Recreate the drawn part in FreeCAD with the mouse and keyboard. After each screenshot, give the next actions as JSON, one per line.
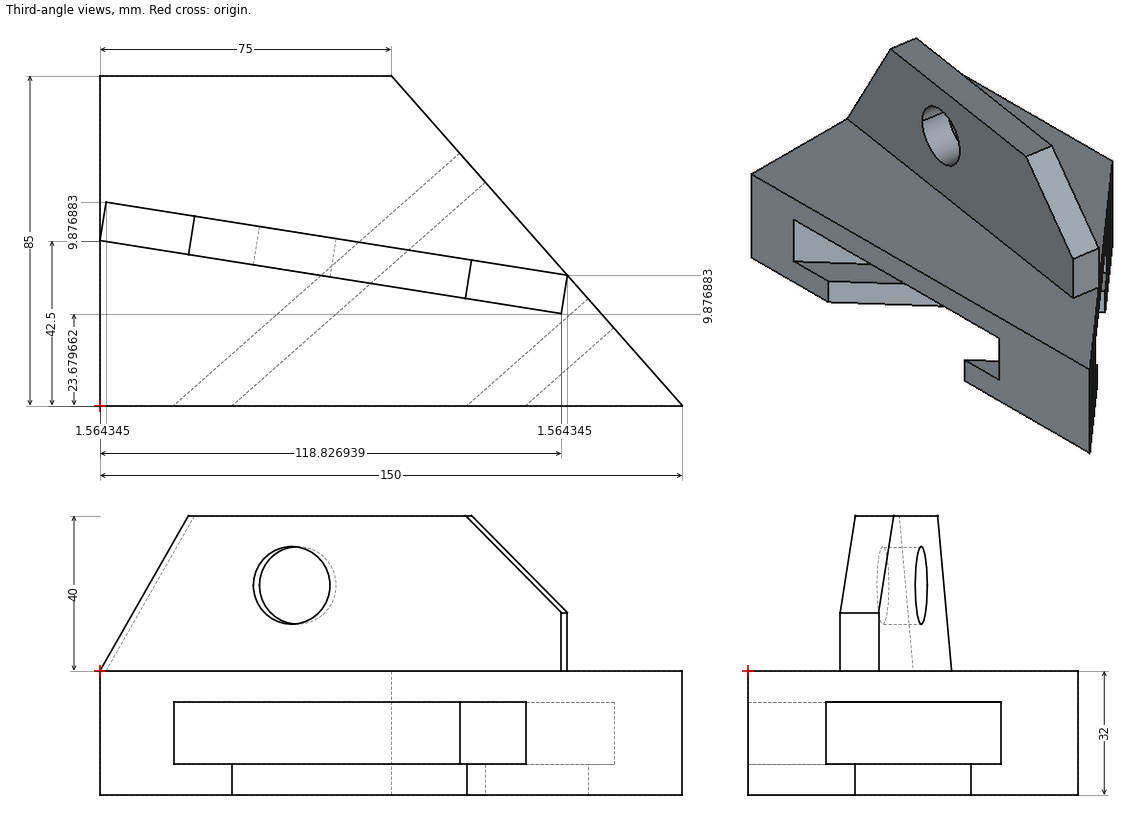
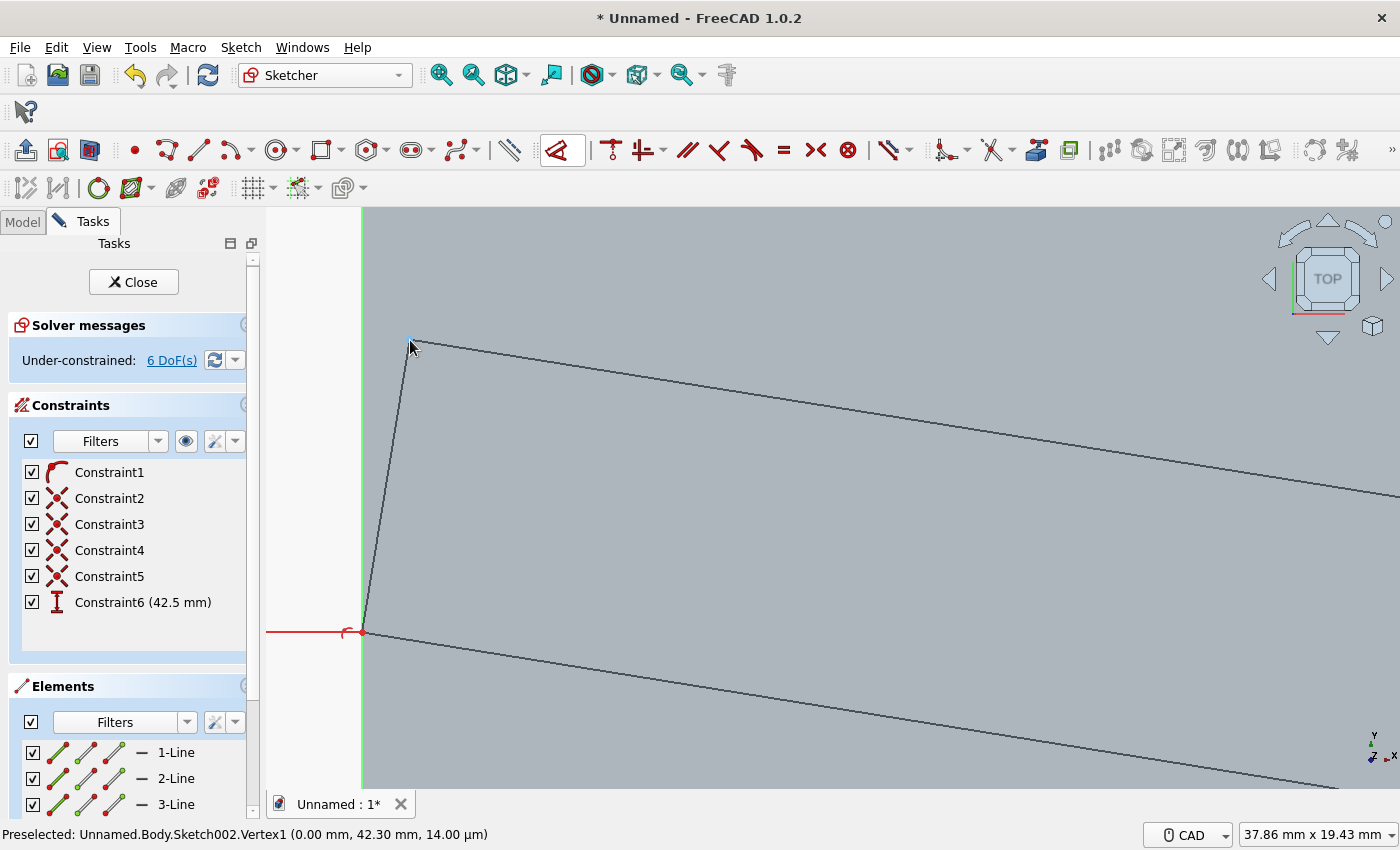
{"action": "left_click", "coordinate": [410, 340]}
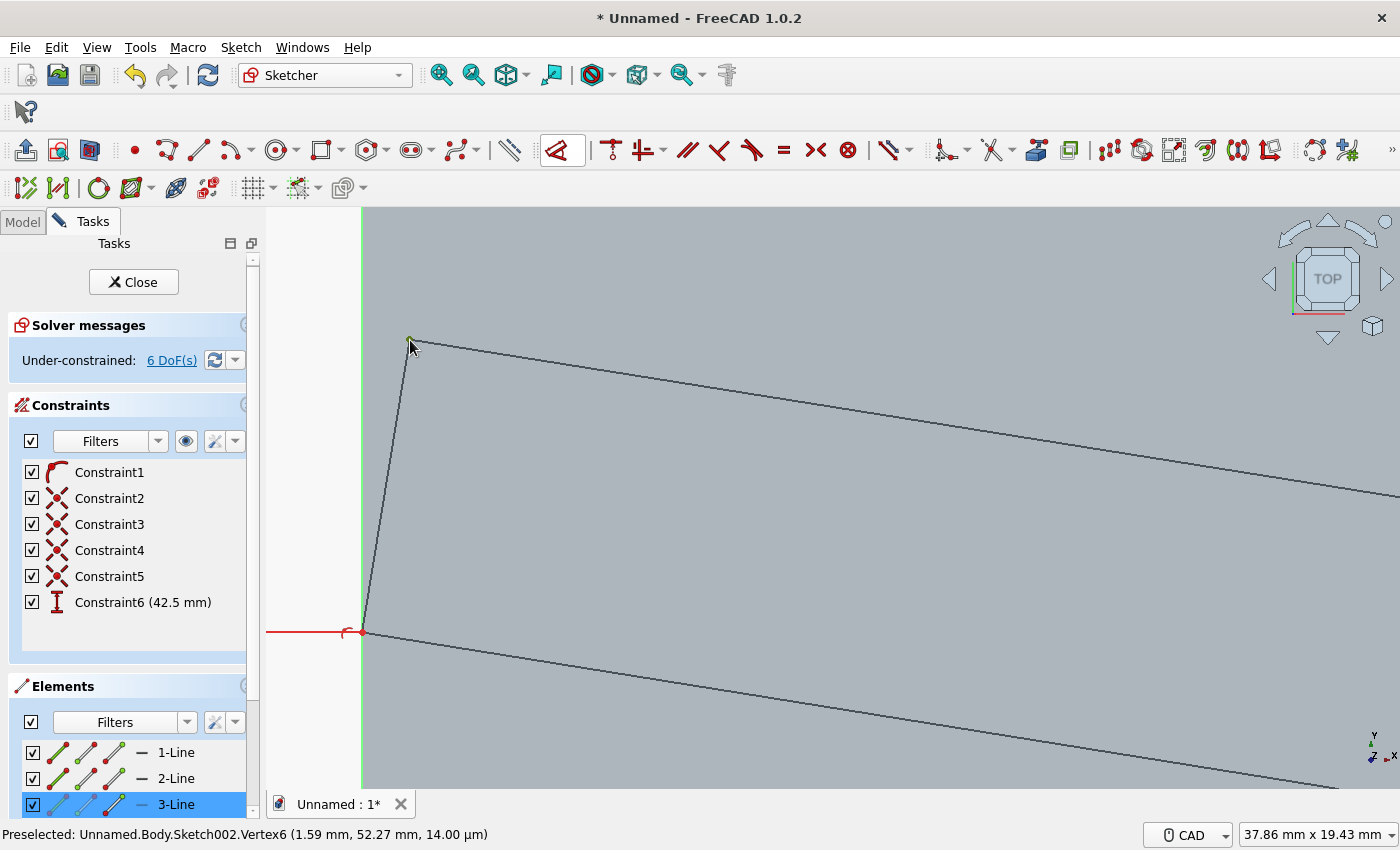
{"action": "key", "text": "l"}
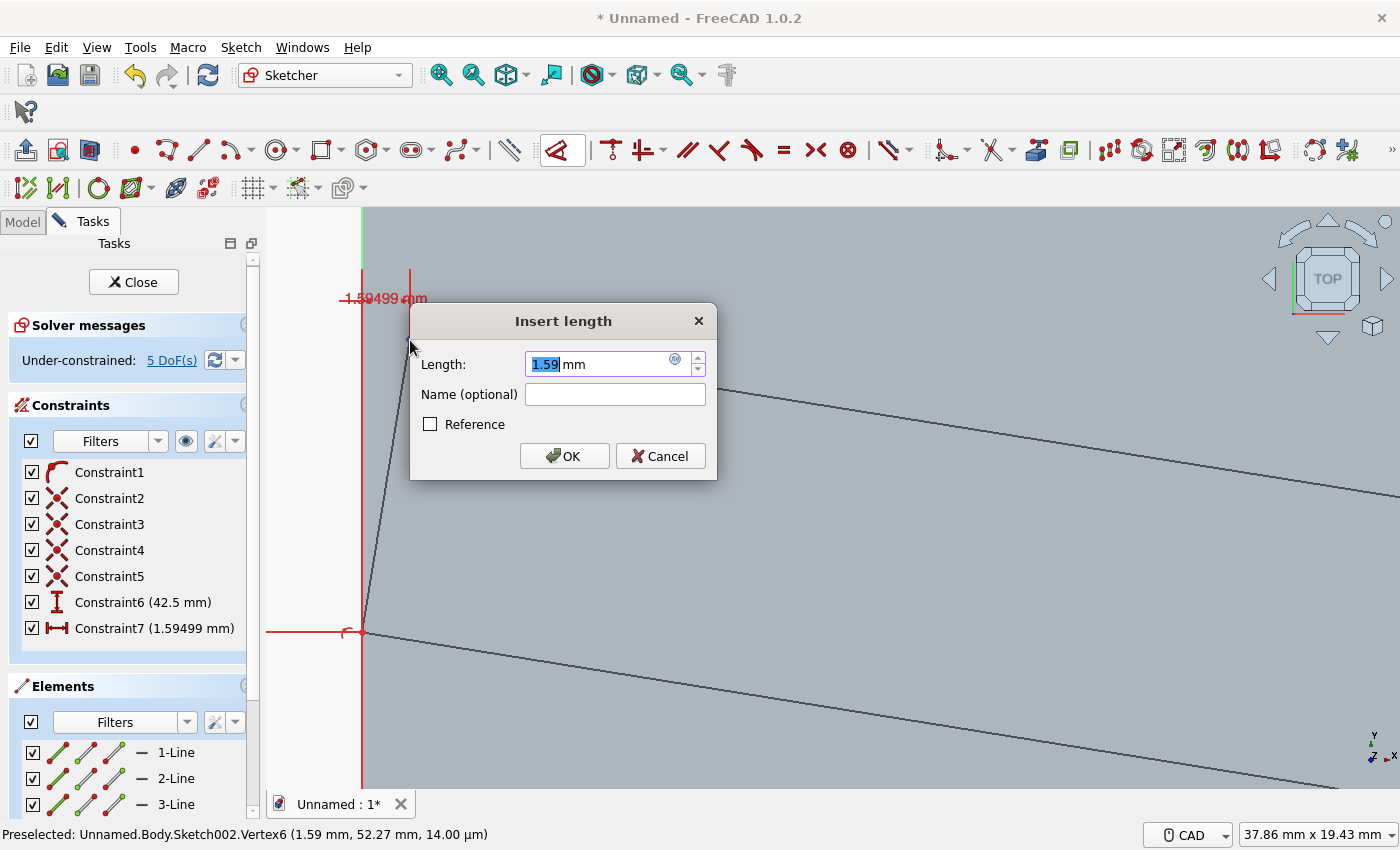
{"action": "type", "text": "1.564345"}
{"action": "key", "text": "Return"}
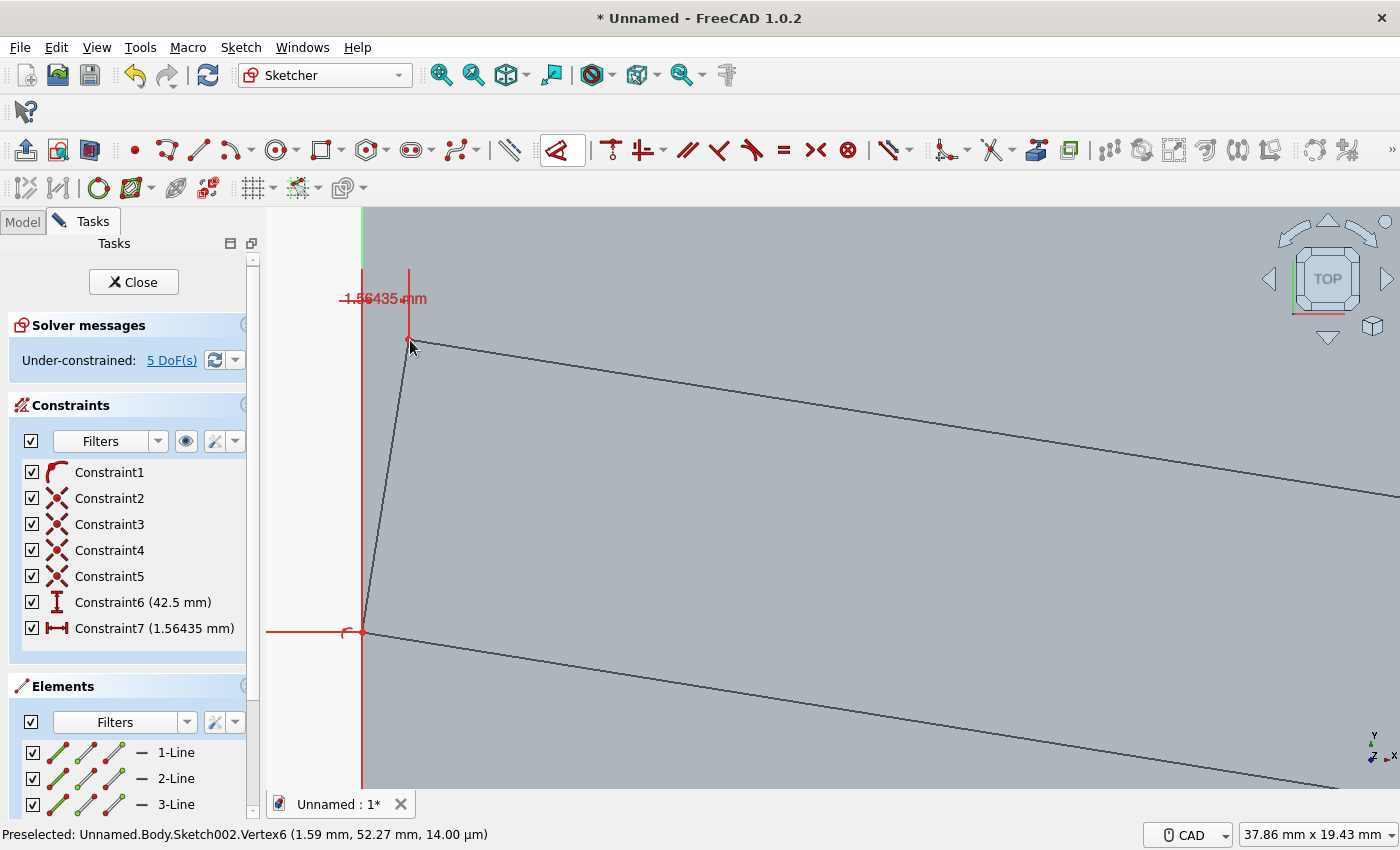
{"action": "scroll", "coordinate": [410, 340], "scroll_direction": "down", "scroll_amount": 8}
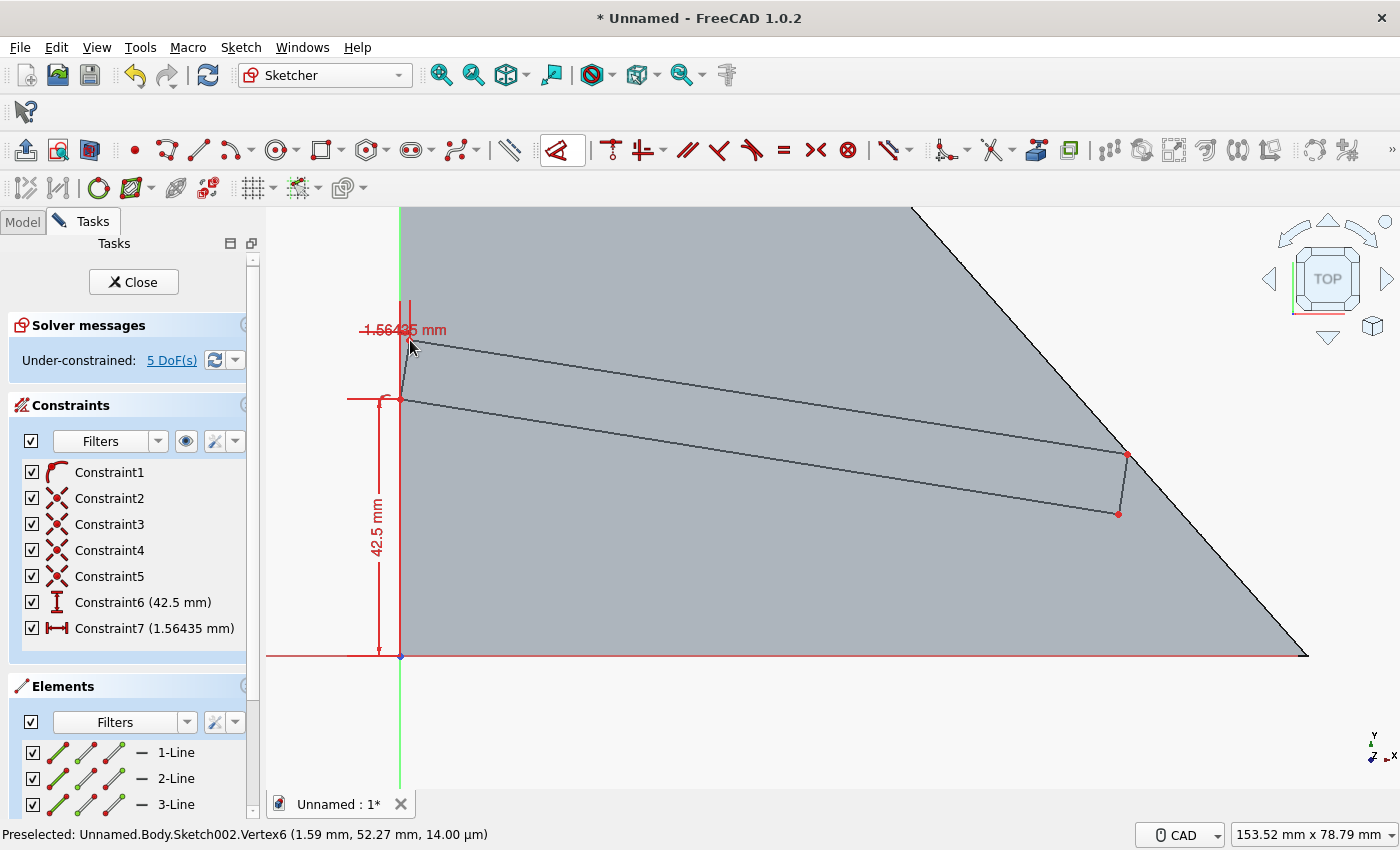
{"action": "scroll", "coordinate": [1122, 496], "scroll_direction": "up", "scroll_amount": 8}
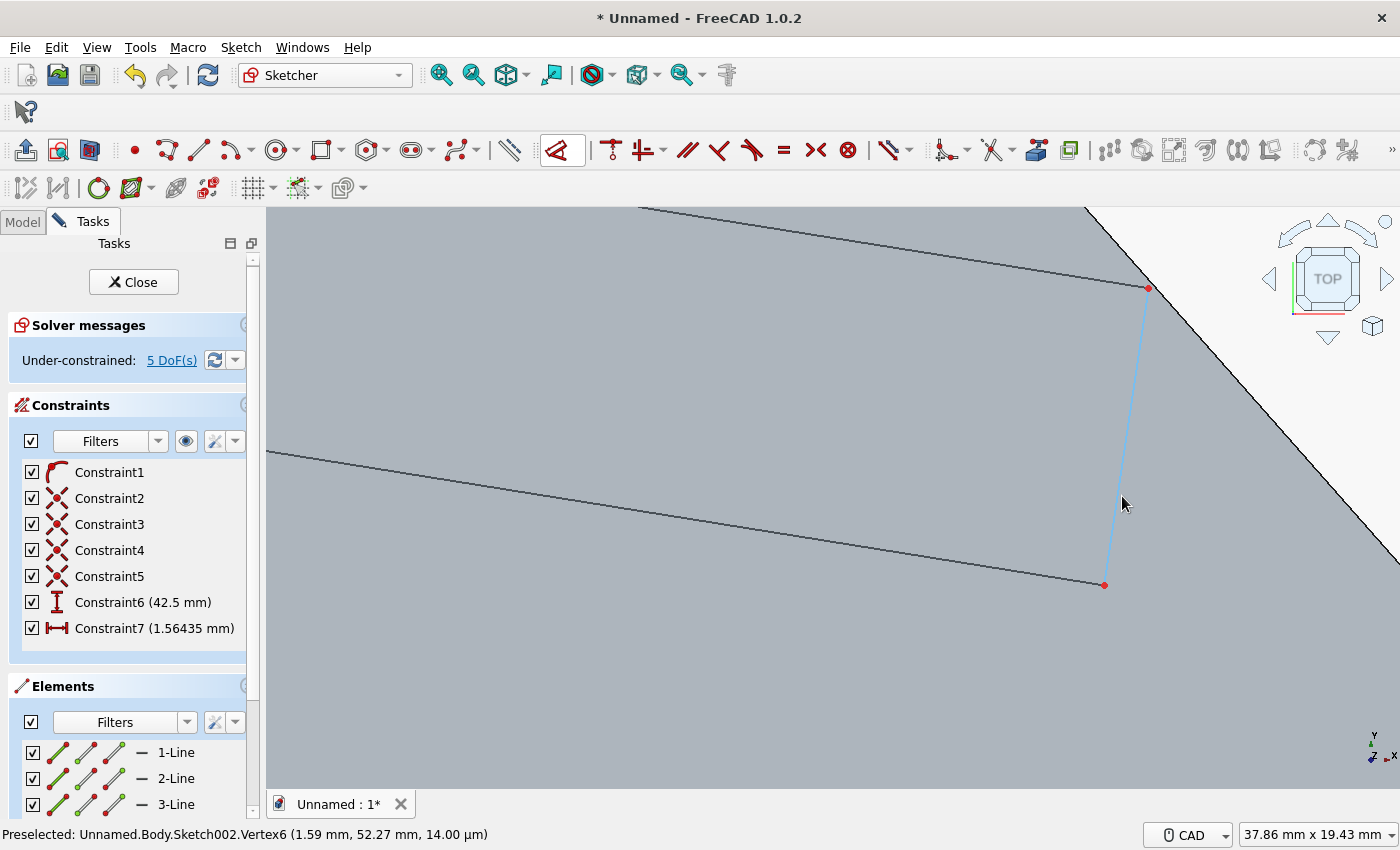
{"action": "left_click", "coordinate": [1118, 496]}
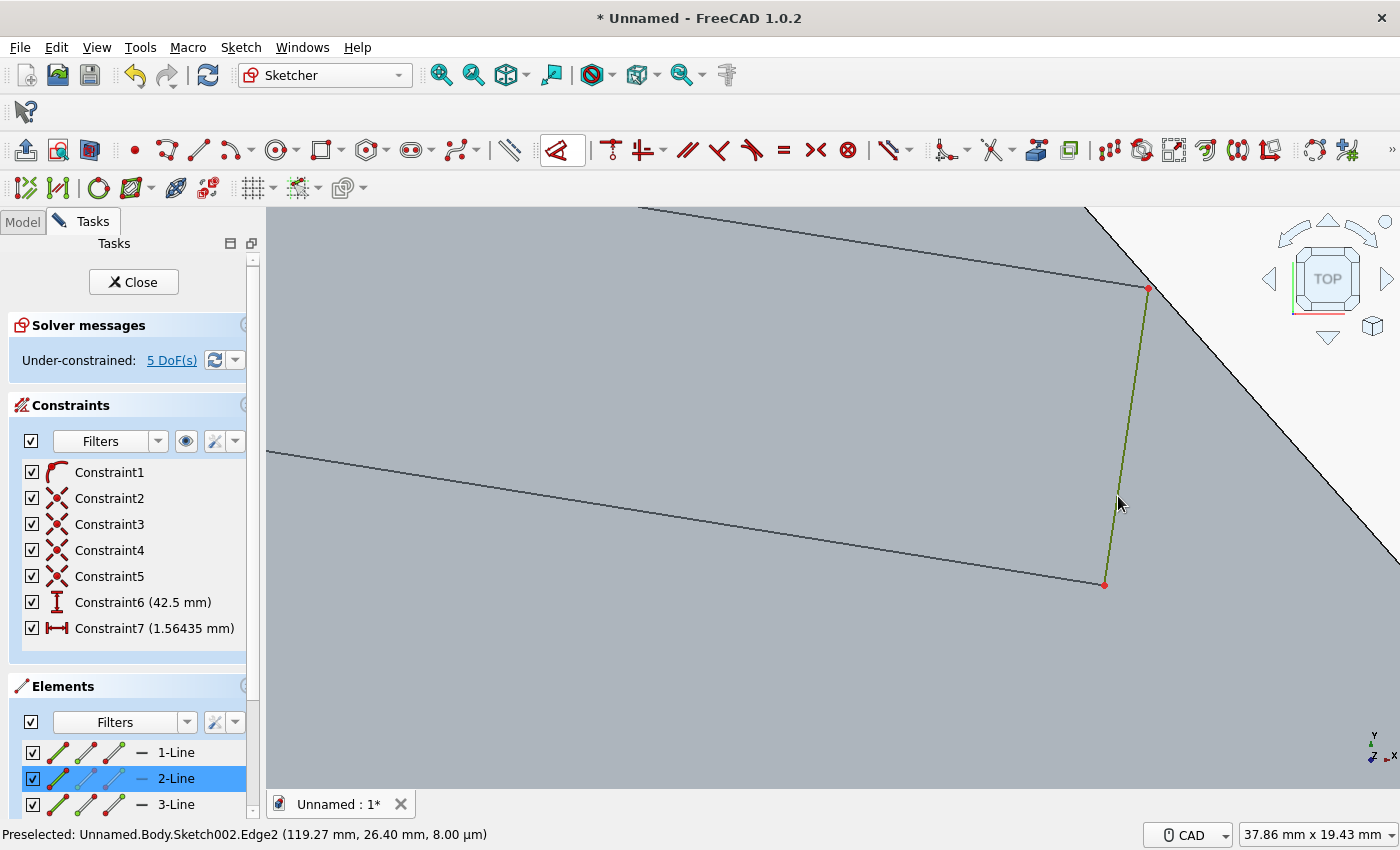
{"action": "key", "text": "l"}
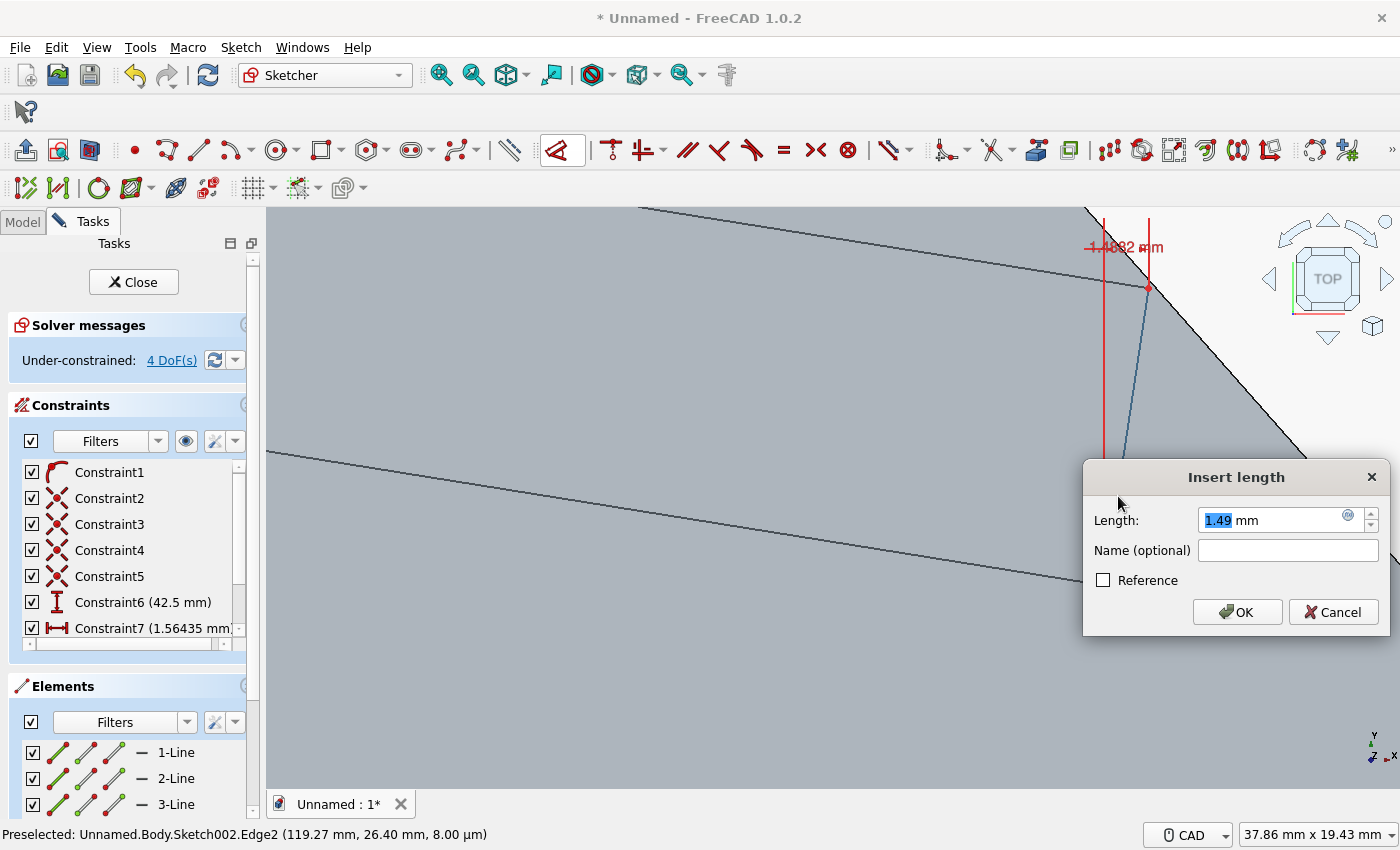
{"action": "type", "text": "1.564345"}
{"action": "key", "text": "Return"}